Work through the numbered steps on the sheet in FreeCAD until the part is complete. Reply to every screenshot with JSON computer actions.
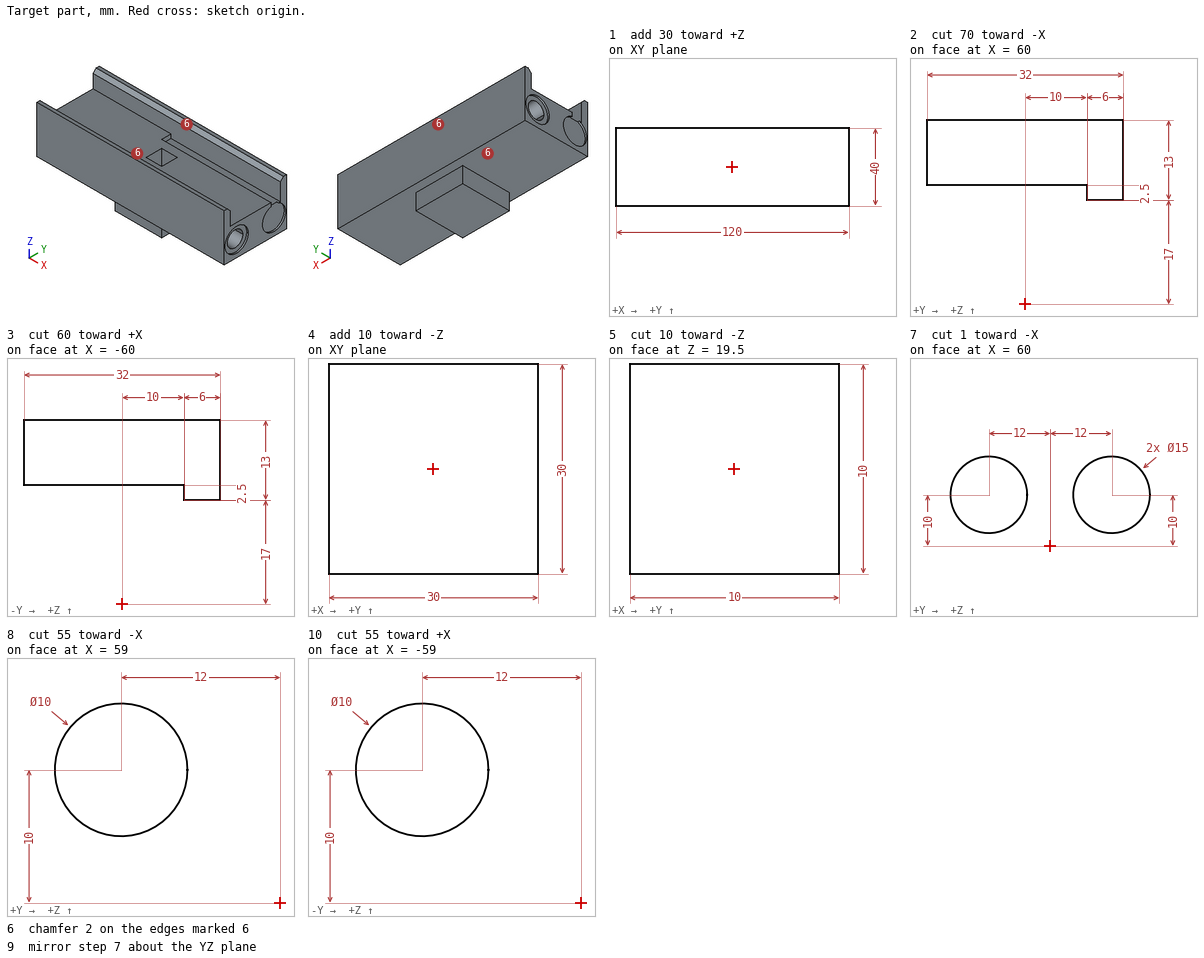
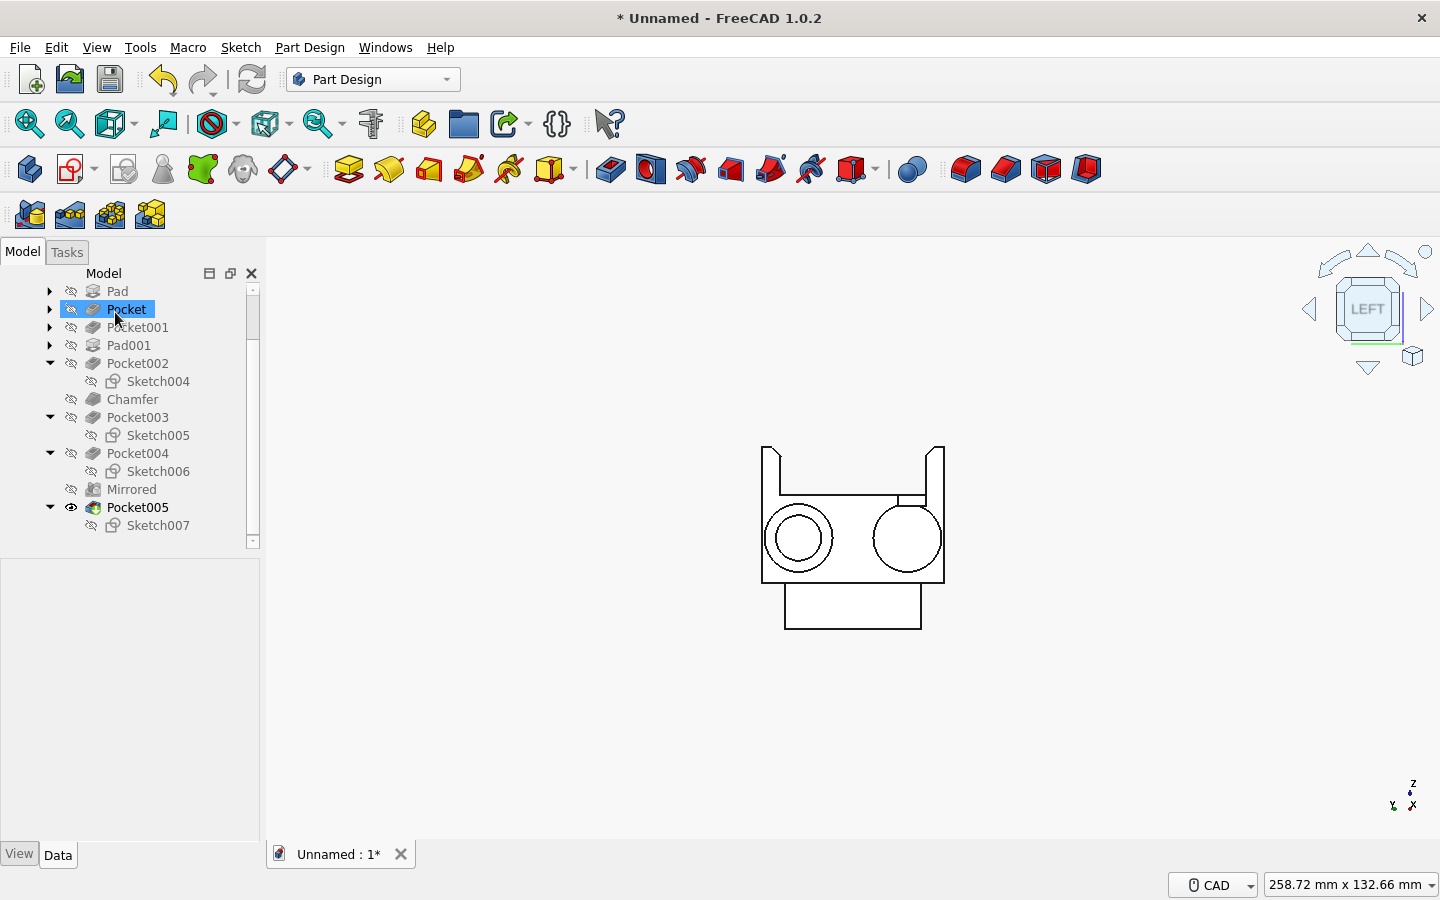
{"action": "key", "text": "0"}